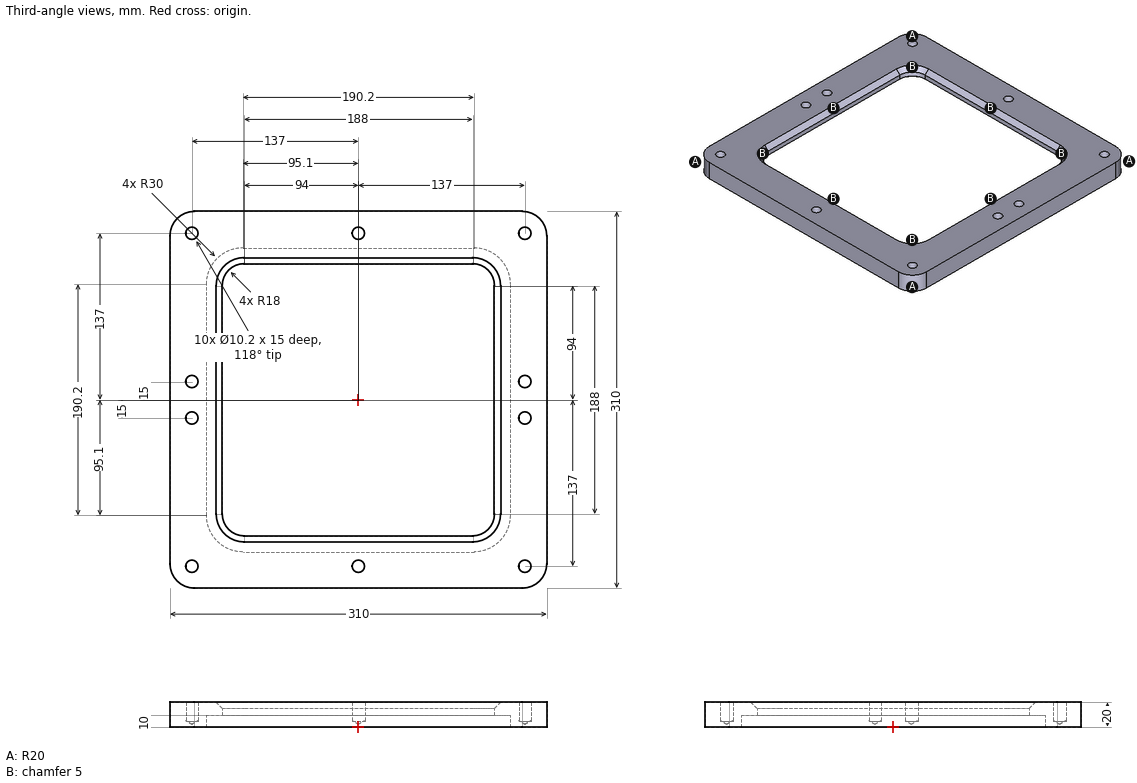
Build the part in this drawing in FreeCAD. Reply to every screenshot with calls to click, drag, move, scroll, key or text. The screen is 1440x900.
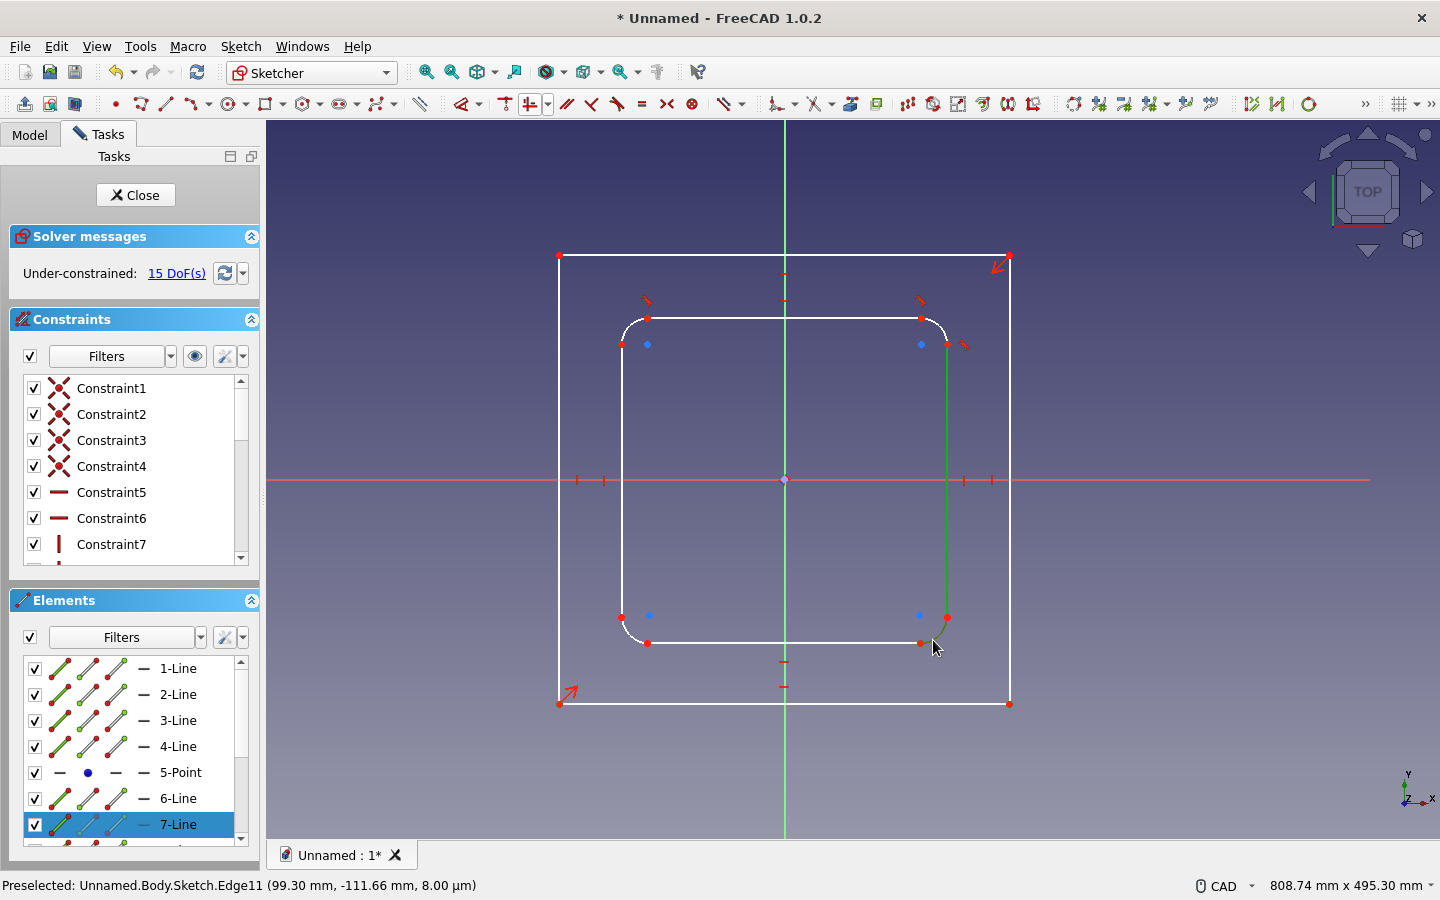
click(617, 104)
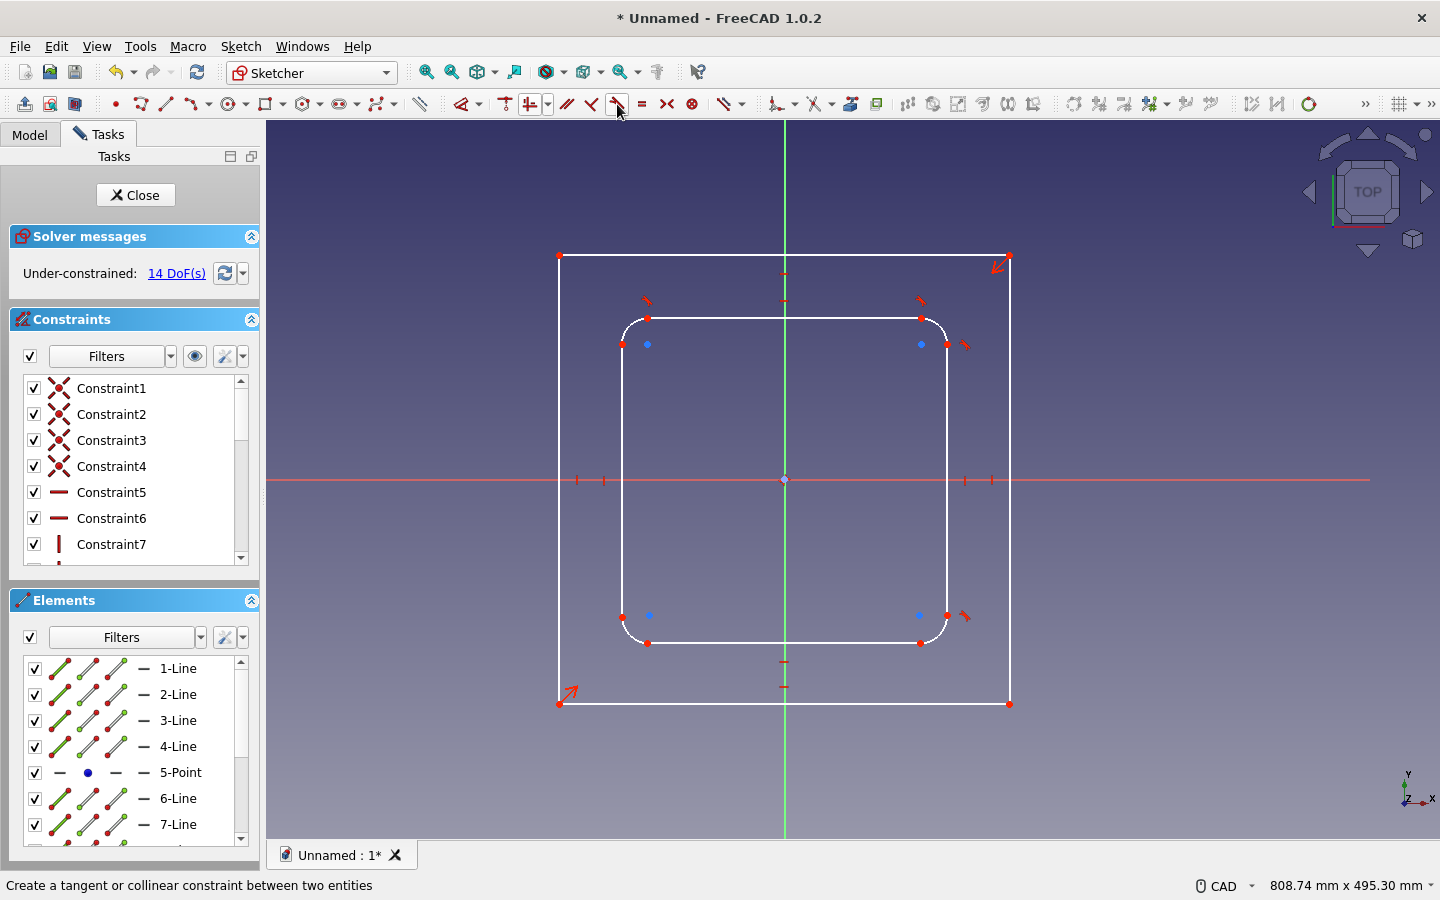
click(839, 643)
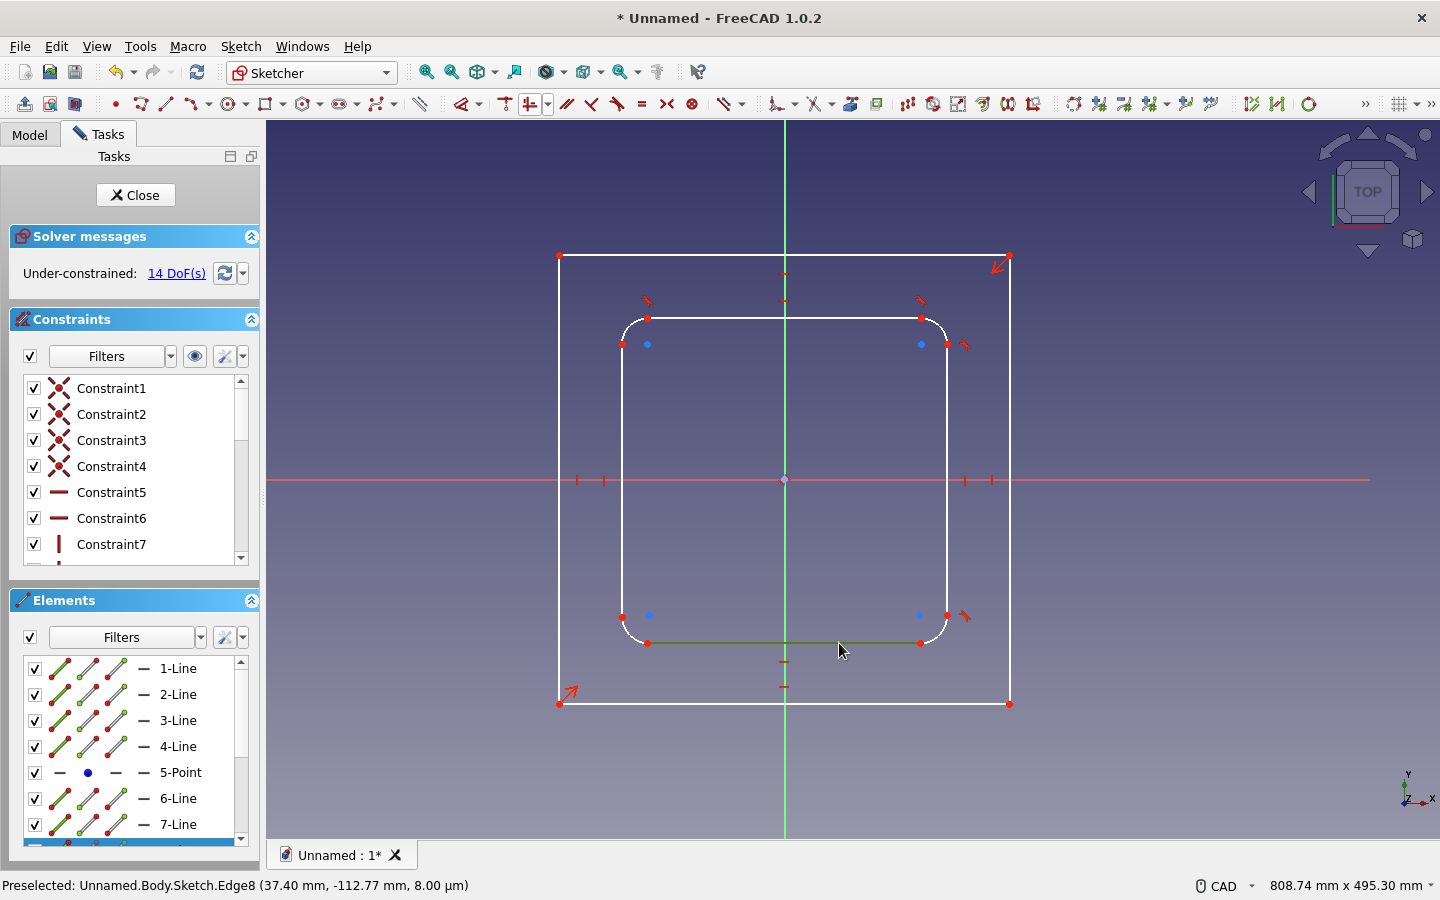
click(933, 640)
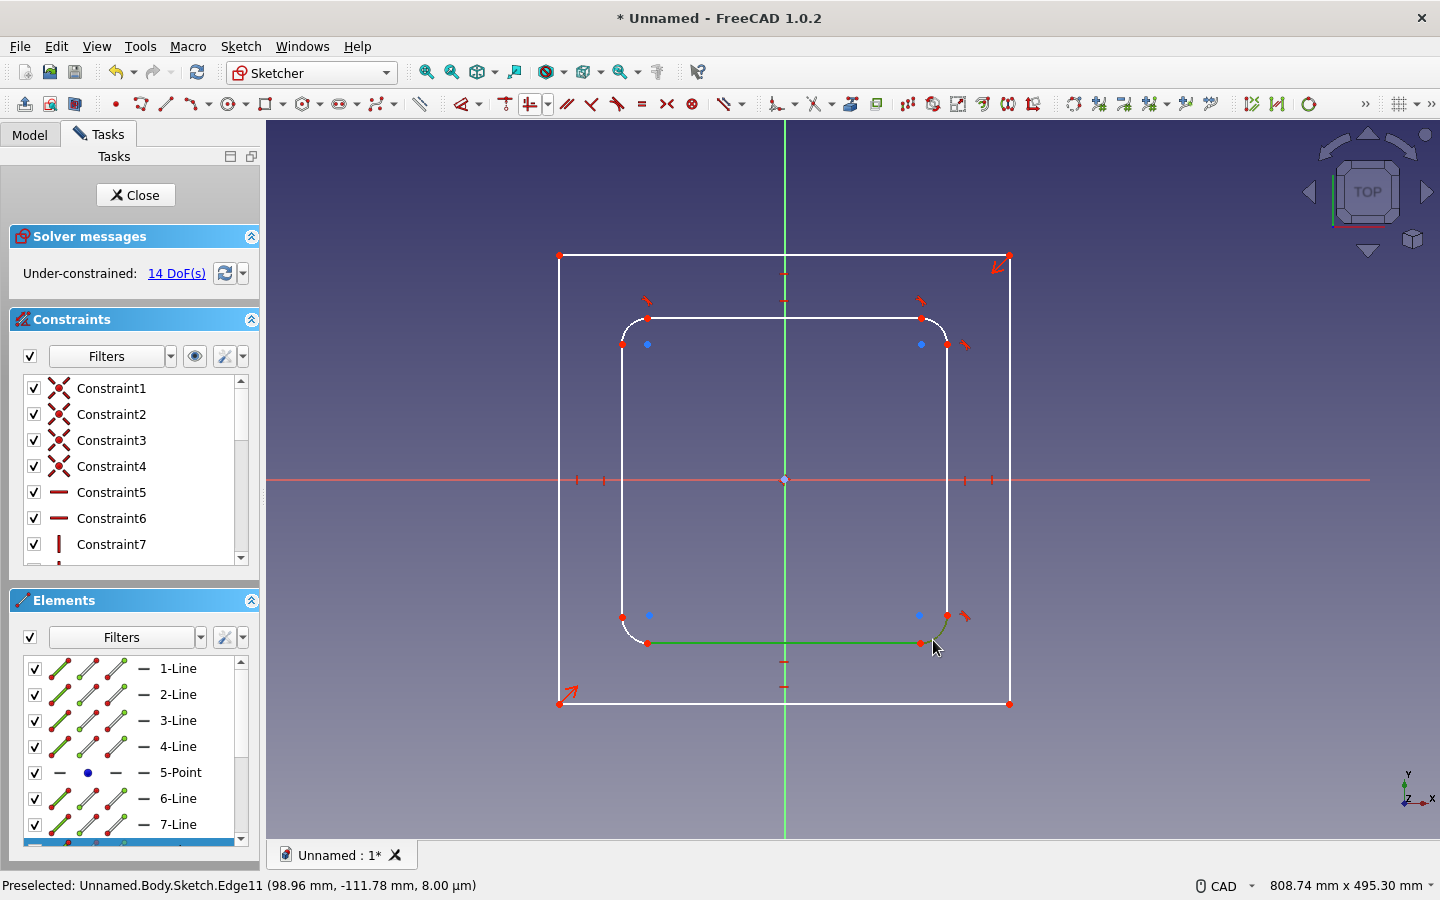
click(617, 104)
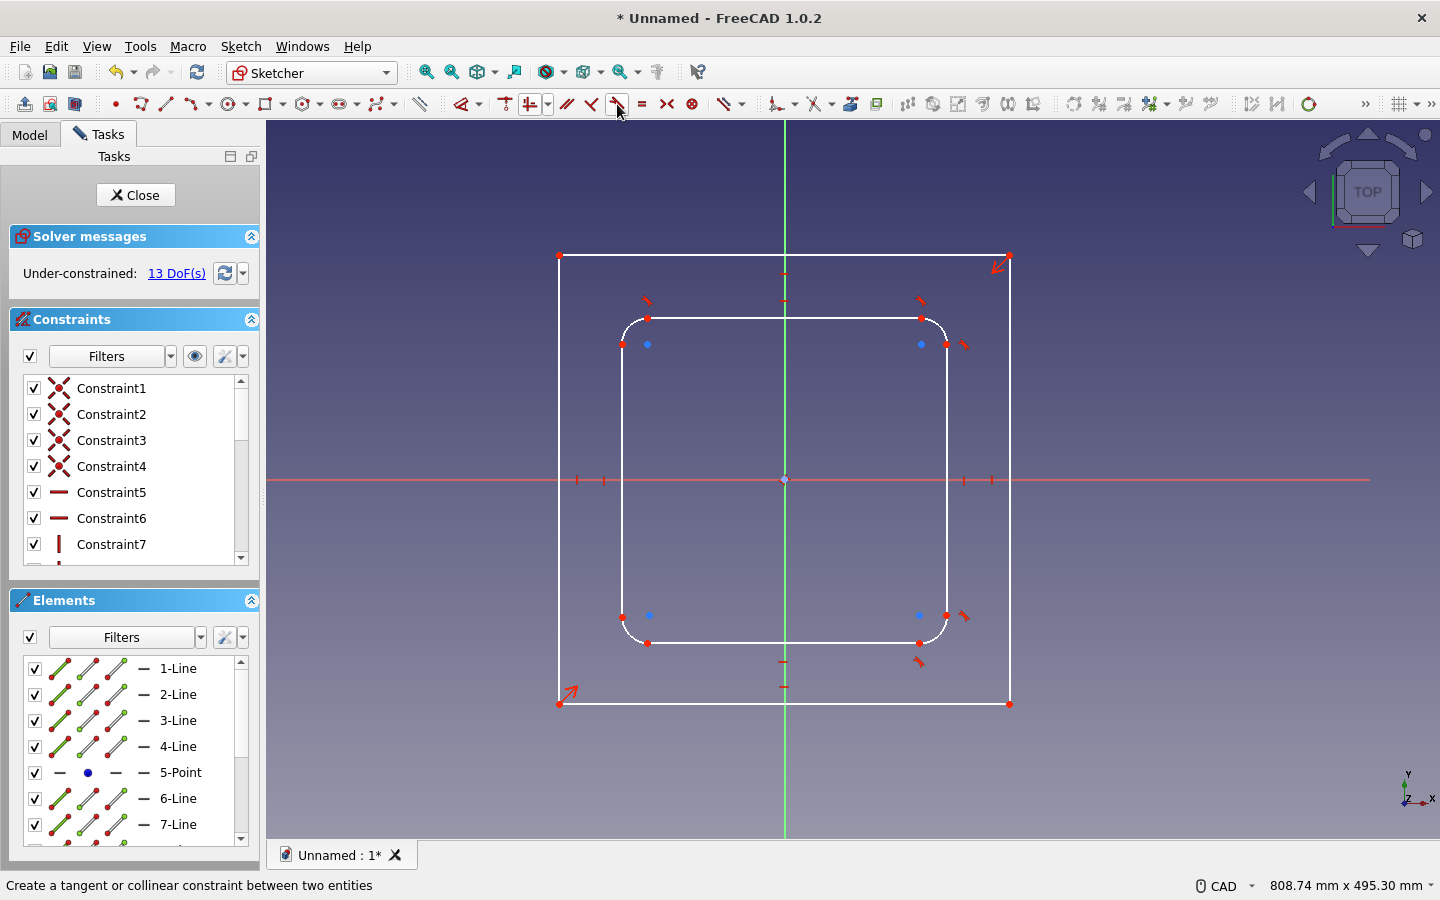
click(838, 643)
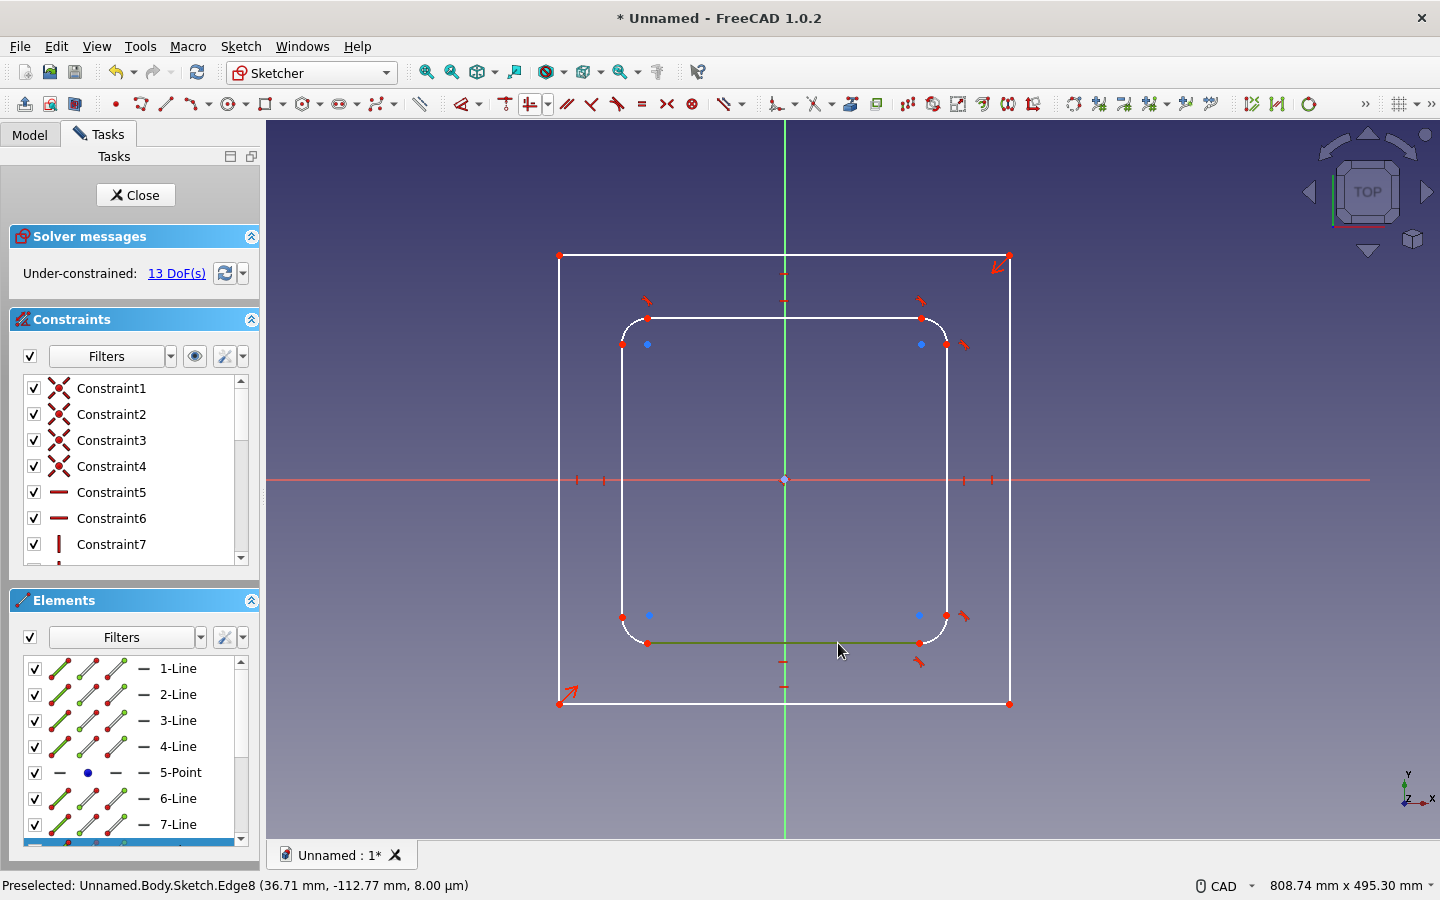
click(625, 629)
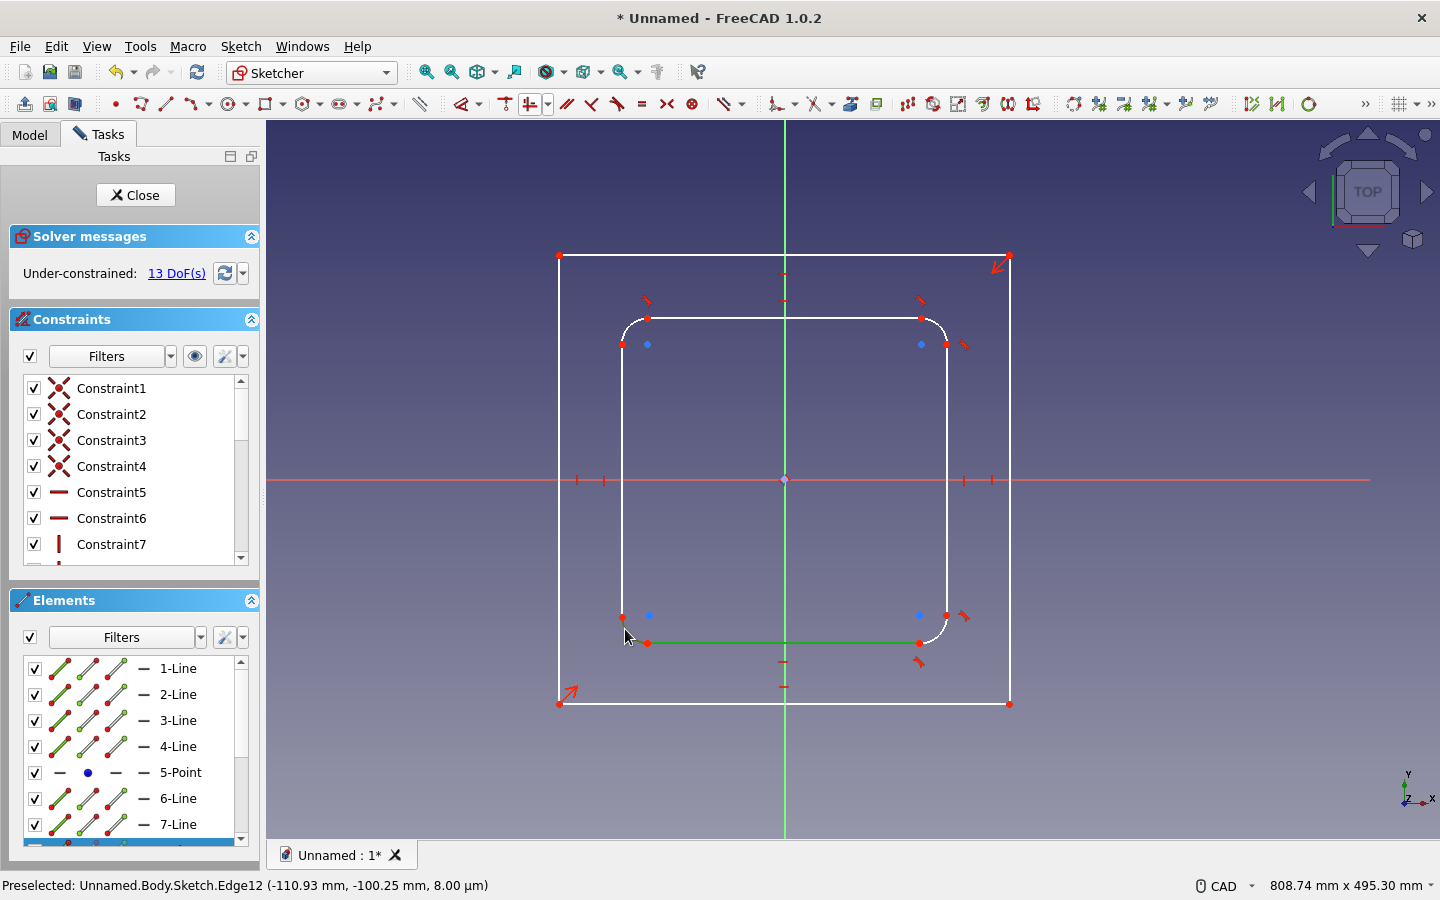
click(617, 104)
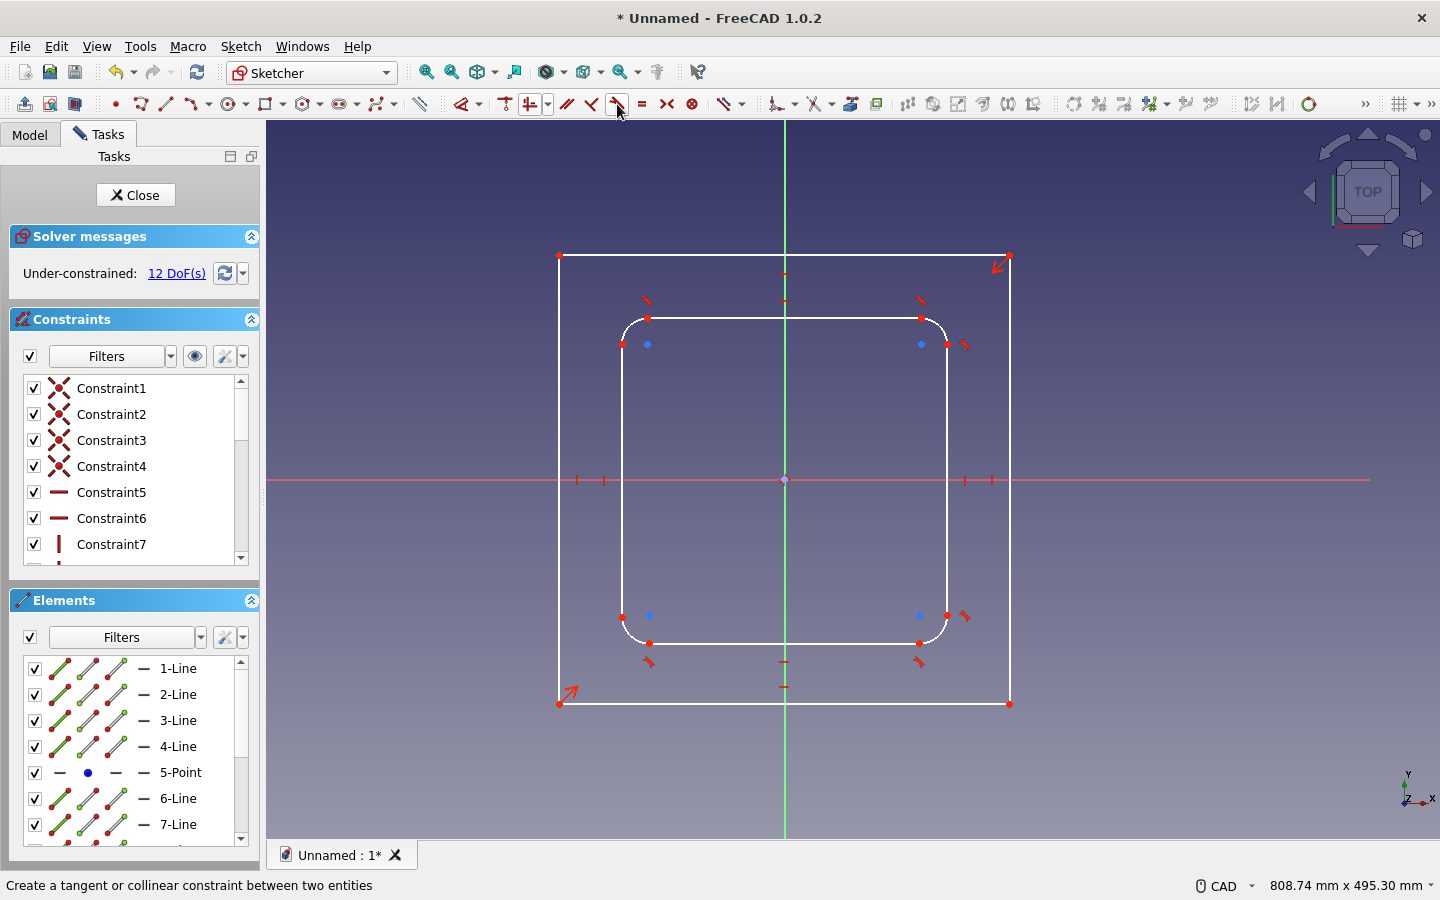
click(622, 536)